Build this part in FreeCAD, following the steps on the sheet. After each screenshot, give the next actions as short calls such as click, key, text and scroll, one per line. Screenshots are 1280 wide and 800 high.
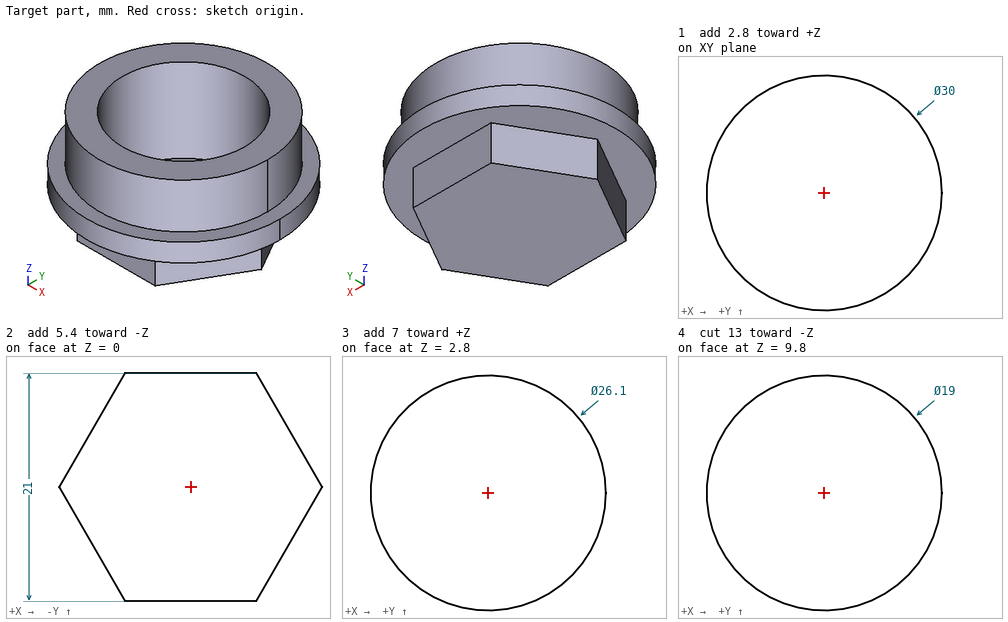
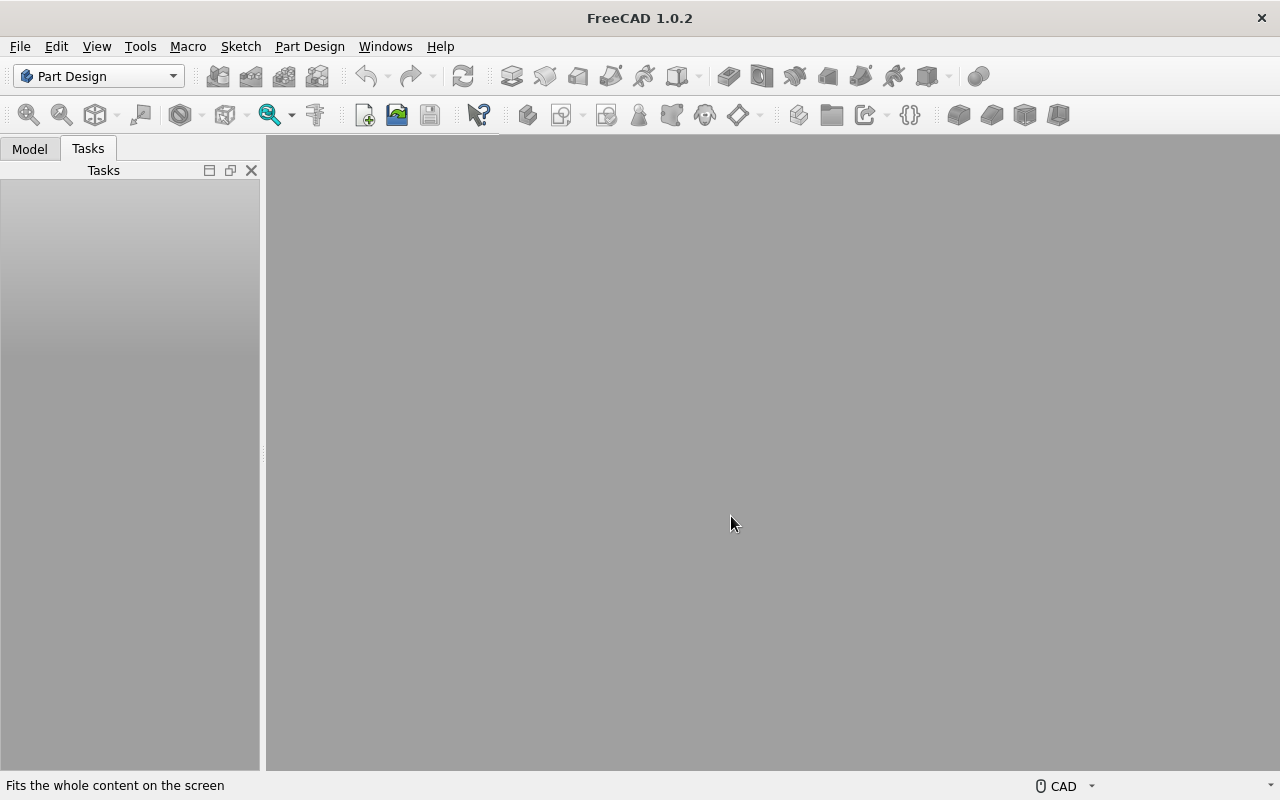
click(364, 116)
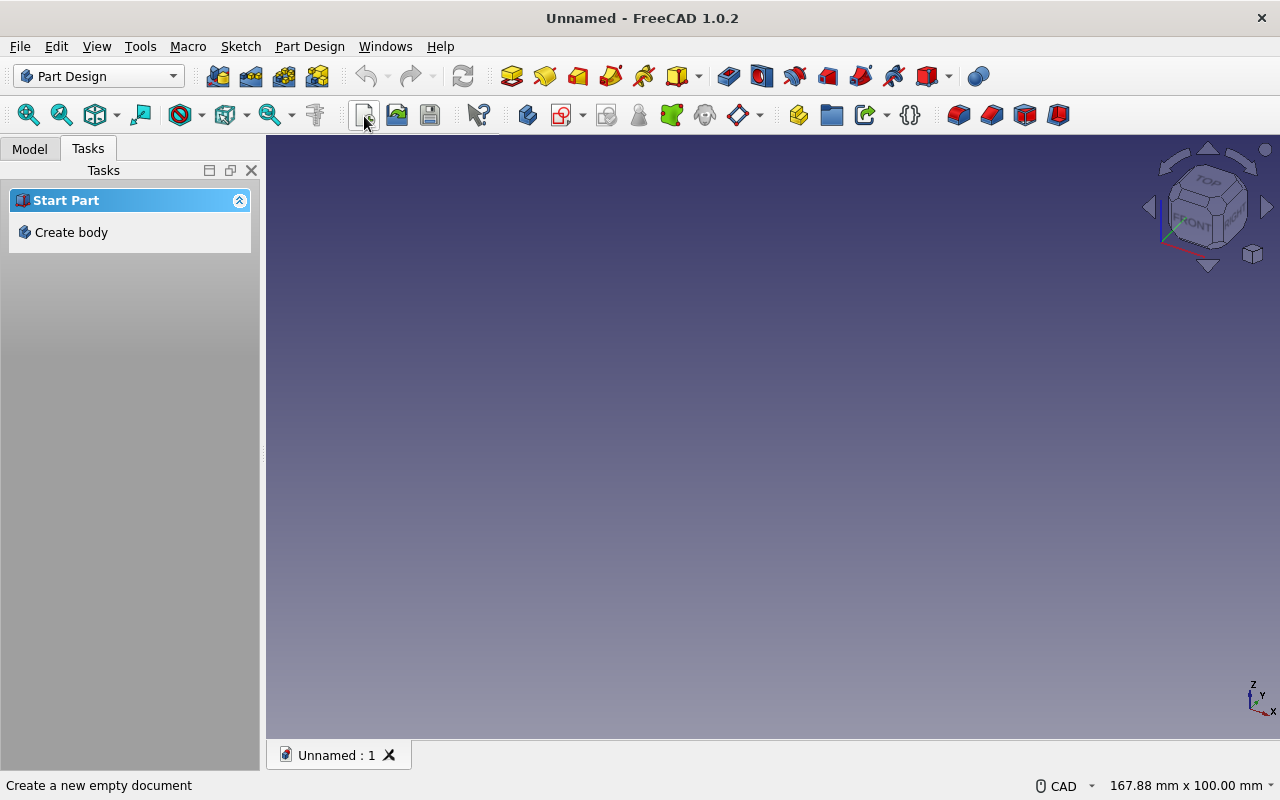
click(560, 116)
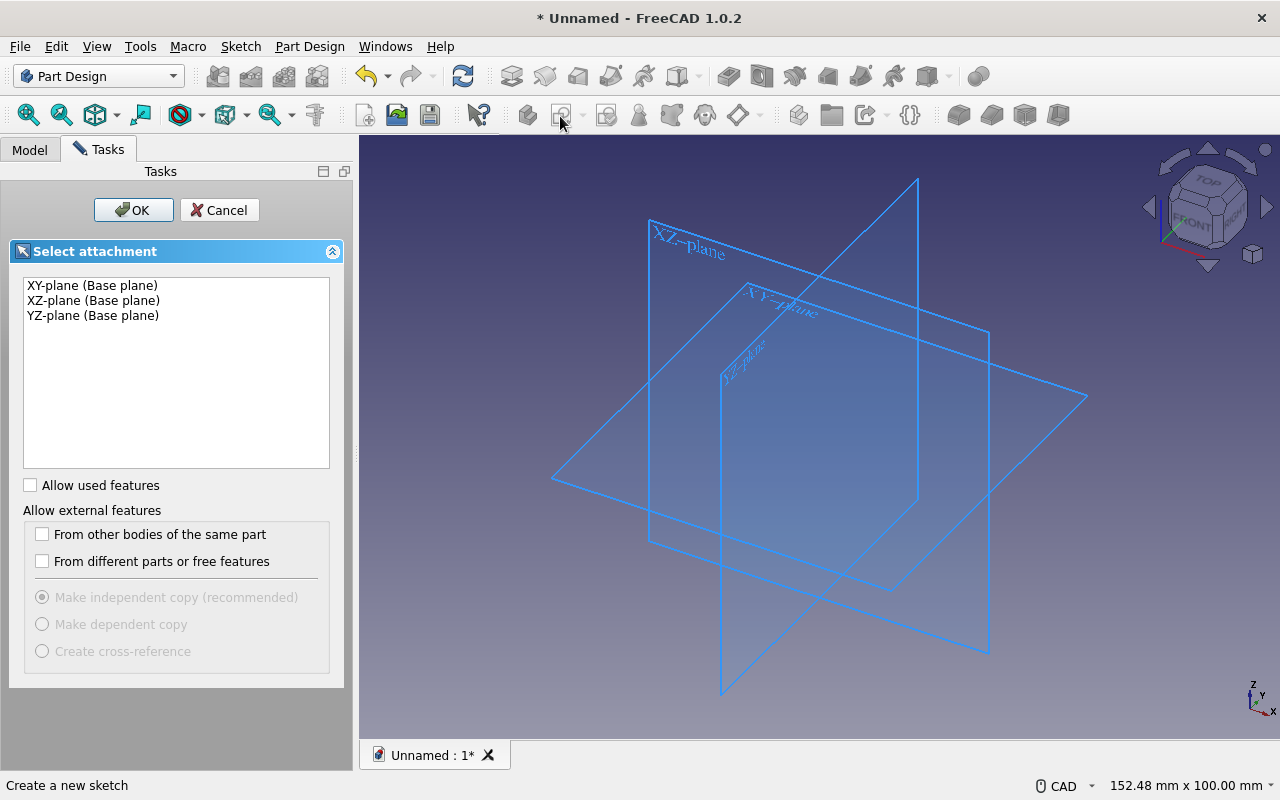
click(84, 286)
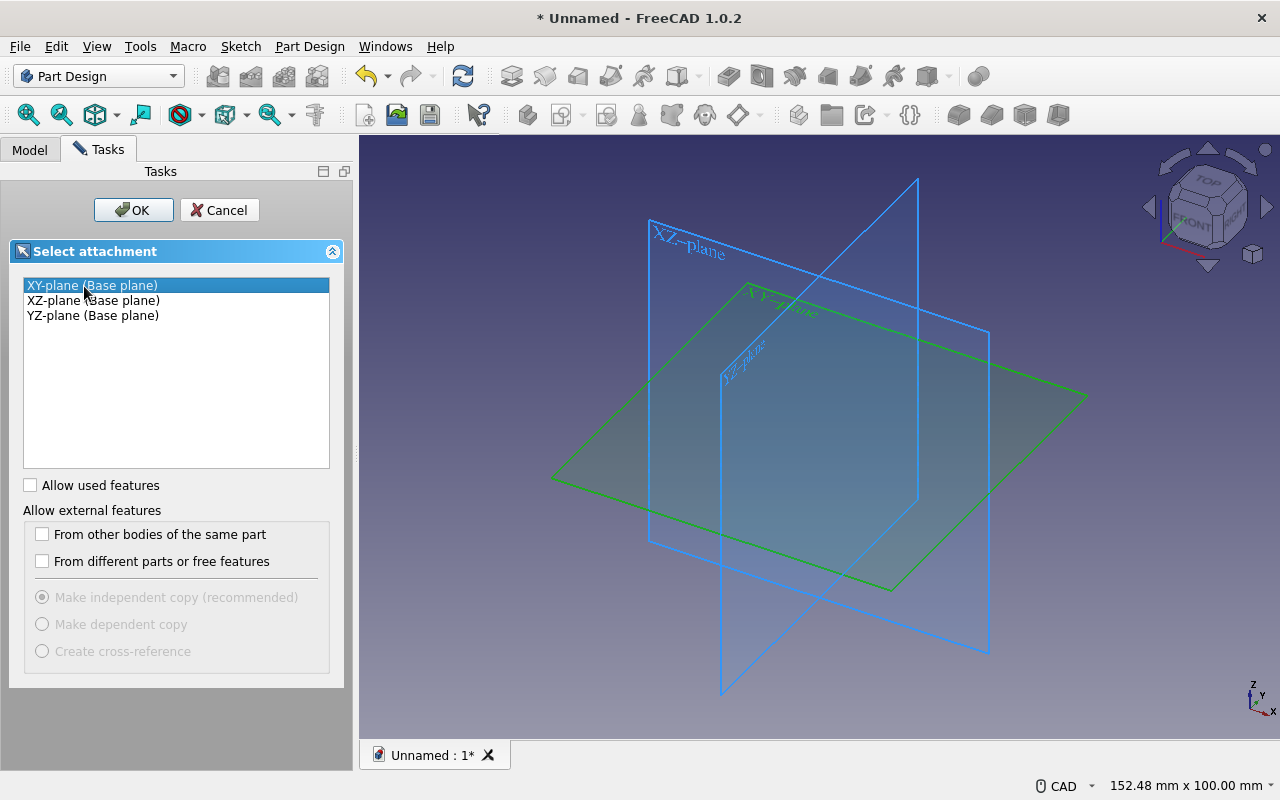
click(134, 210)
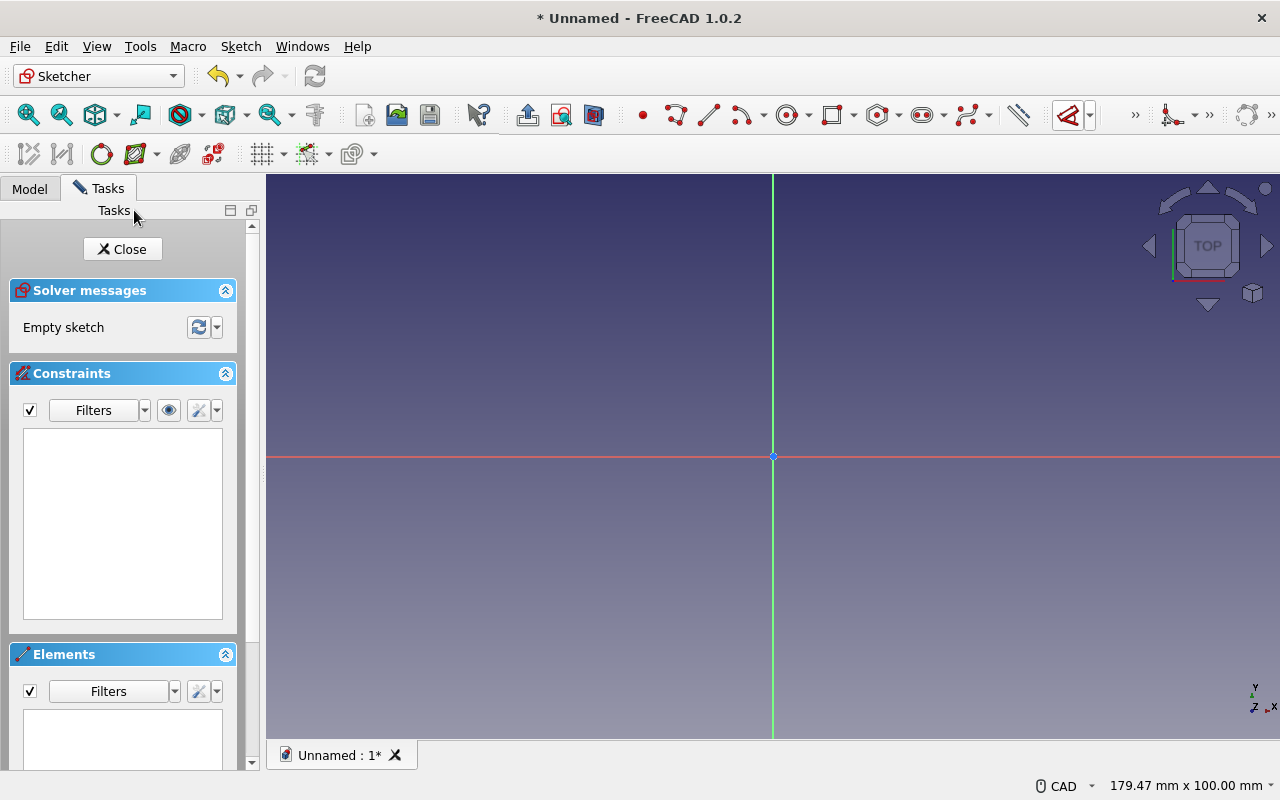
scroll(829, 456, up, 4)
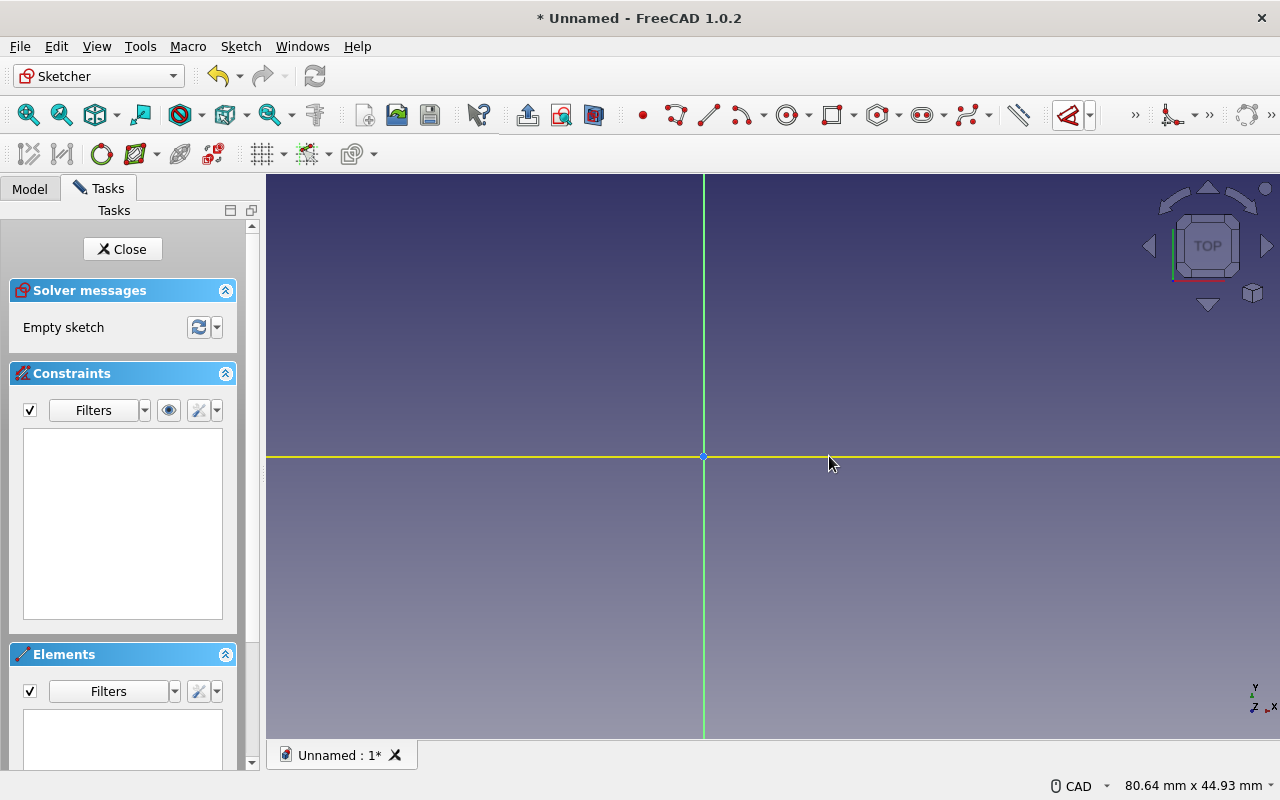
click(786, 116)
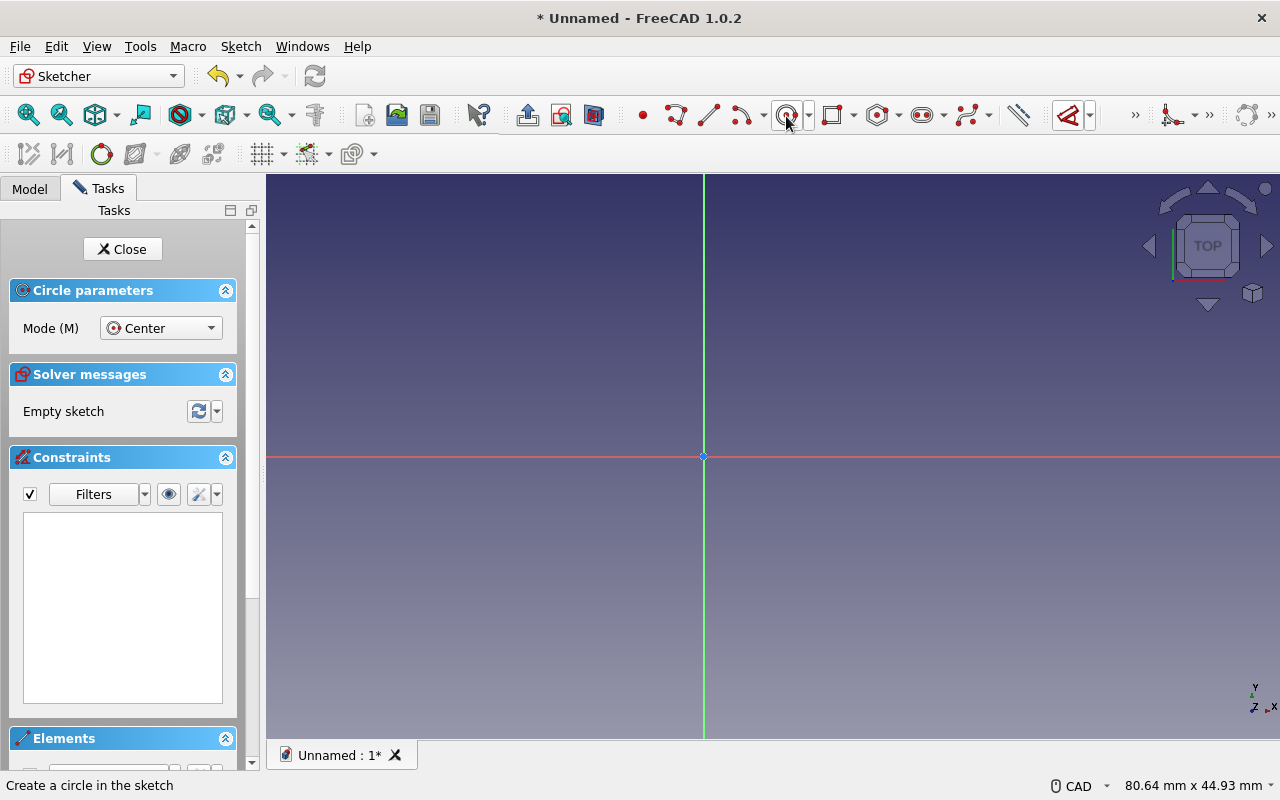
click(704, 456)
move(837, 323)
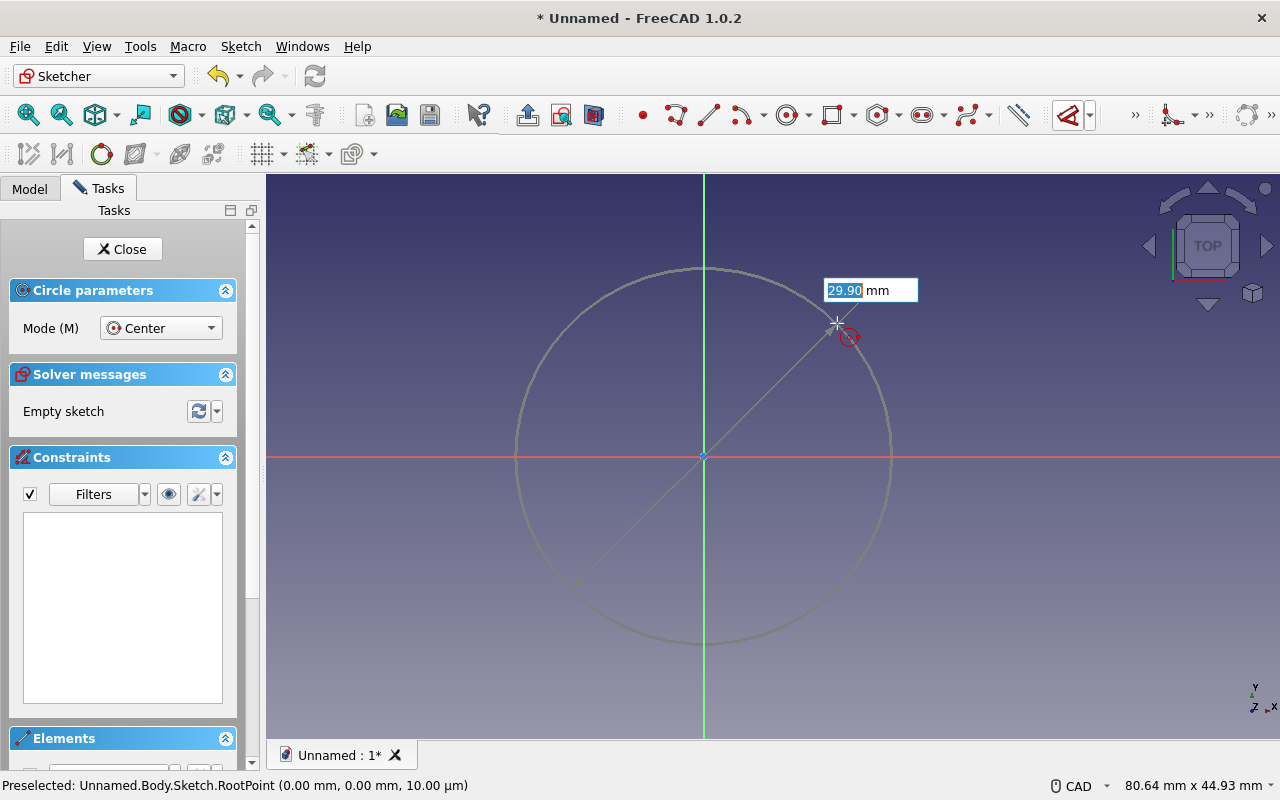
text(30)
key(Return)
key(Escape)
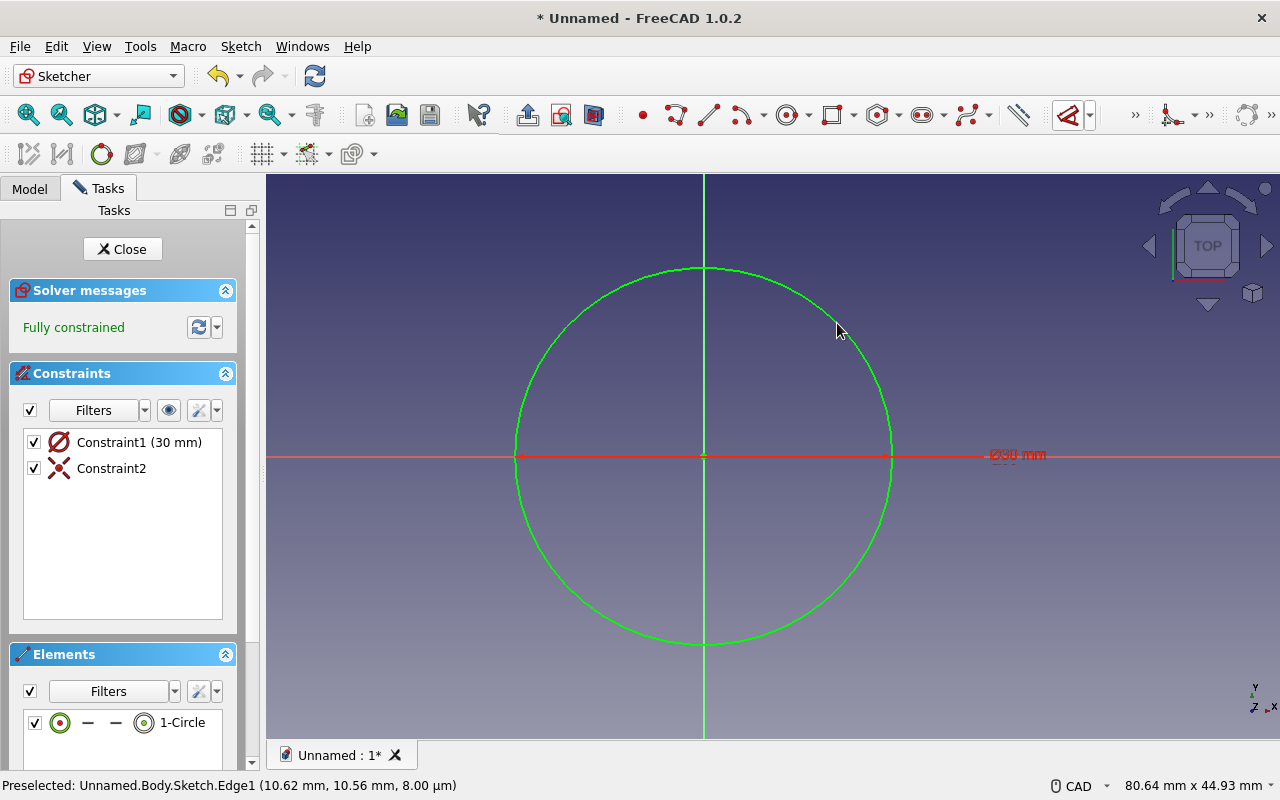
click(123, 249)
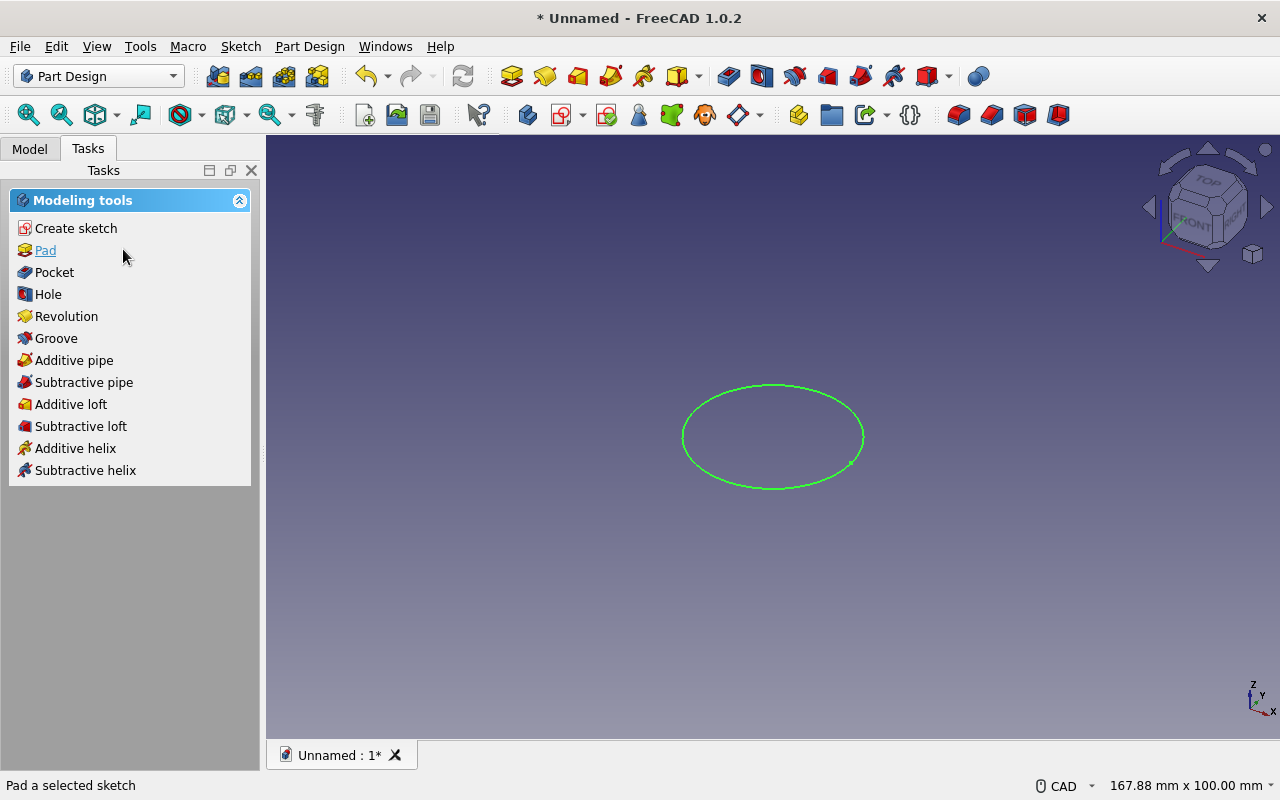
click(512, 76)